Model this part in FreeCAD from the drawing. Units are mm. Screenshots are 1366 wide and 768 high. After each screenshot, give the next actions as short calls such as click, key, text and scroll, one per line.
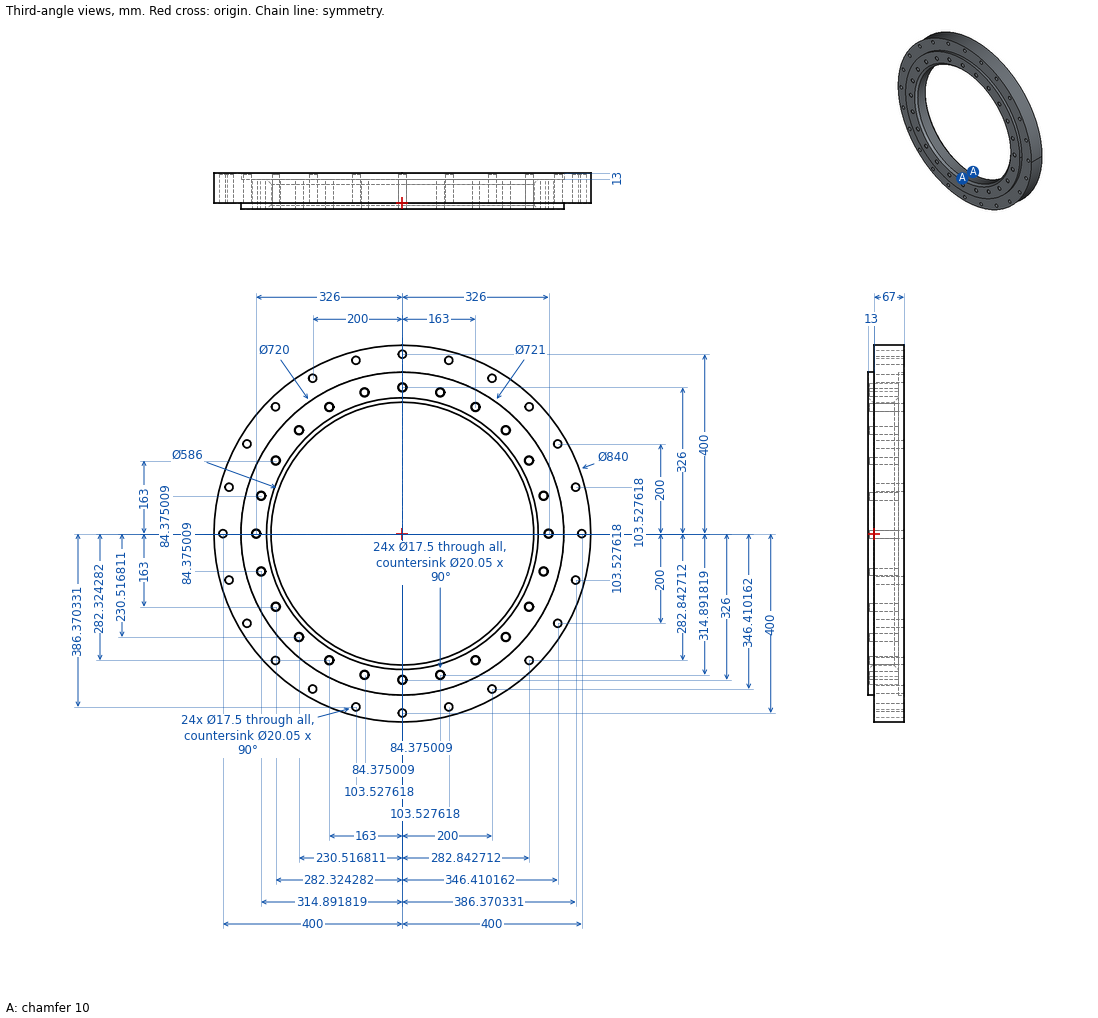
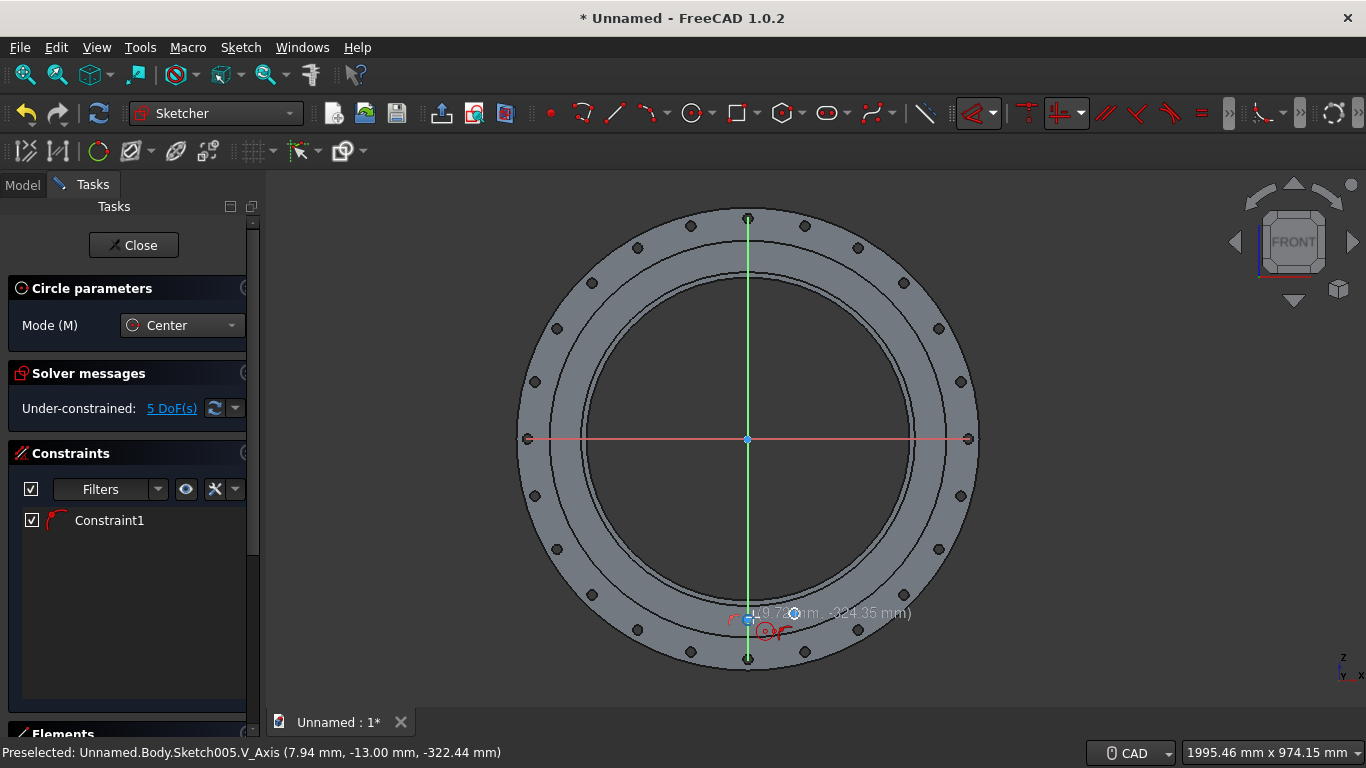
click(701, 613)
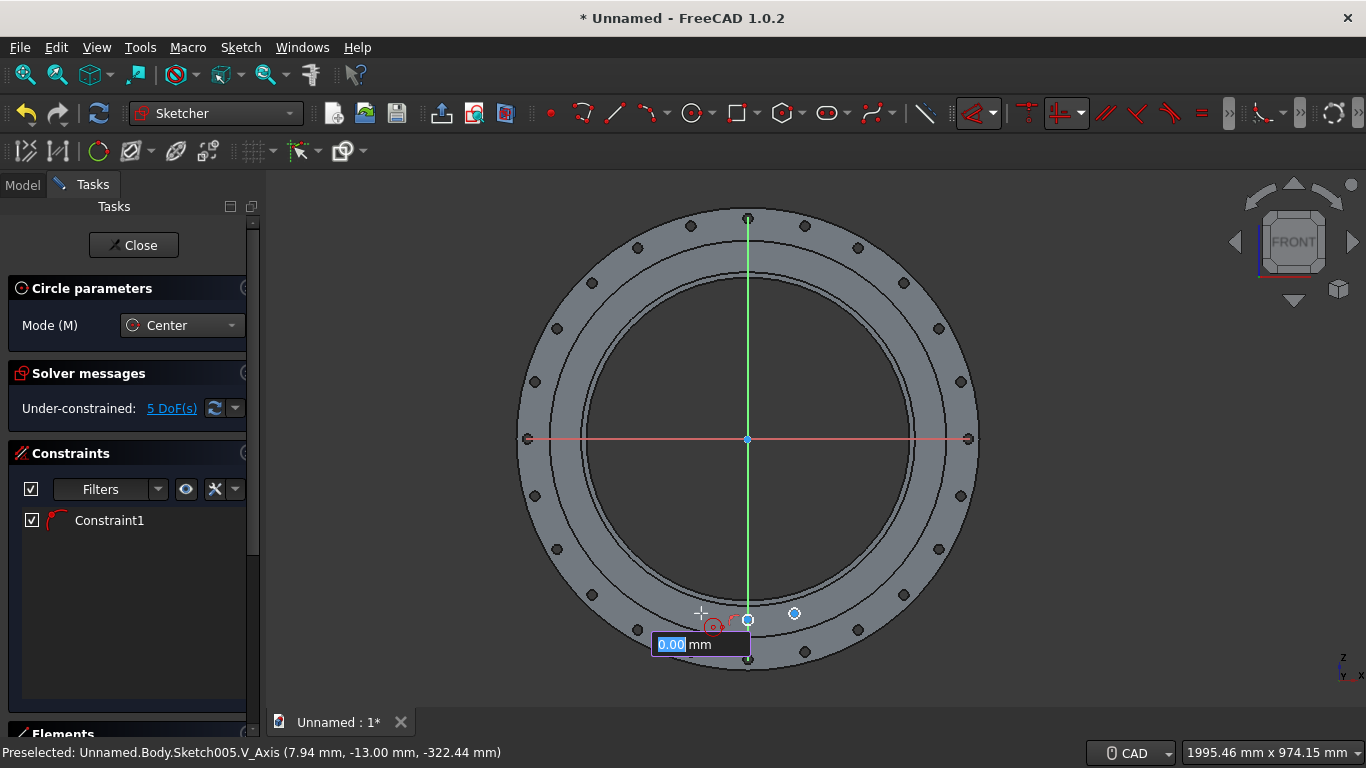
scroll(705, 609, up, 6)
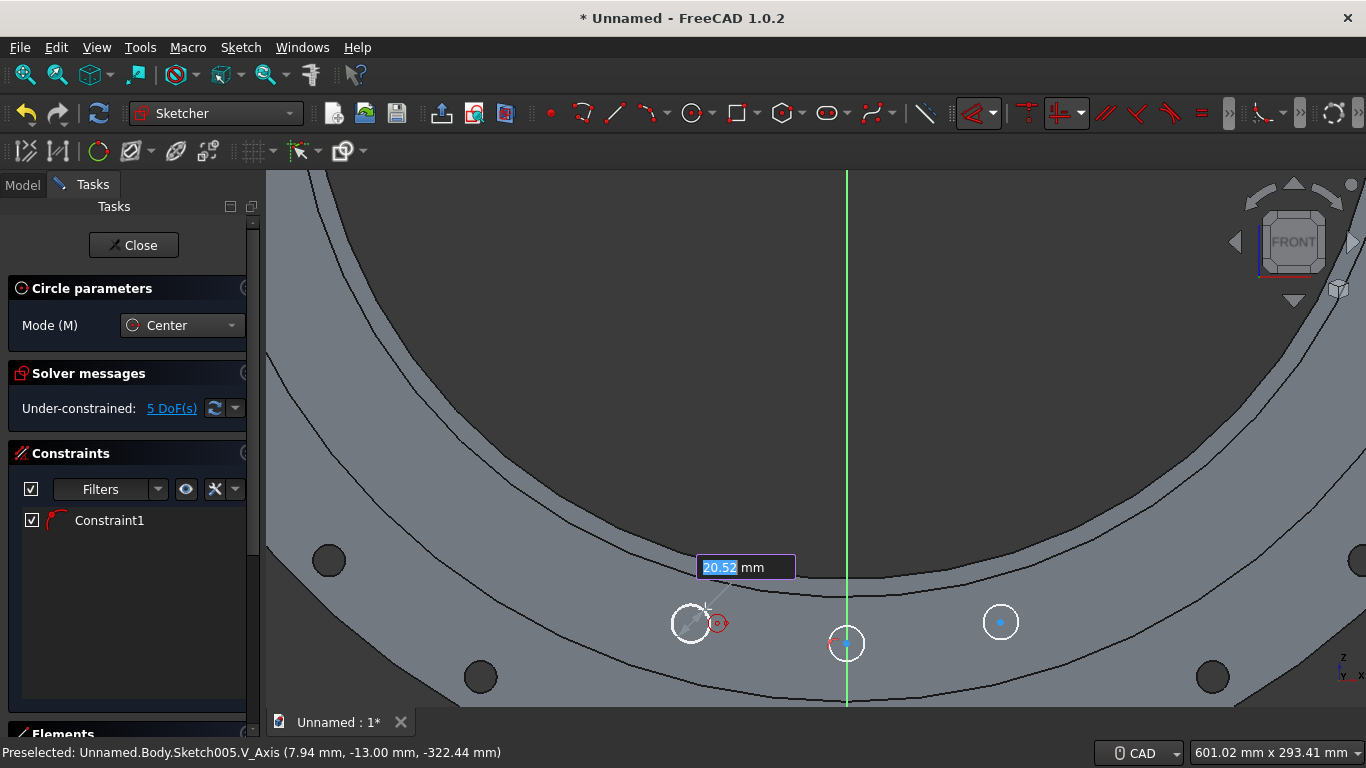
click(704, 608)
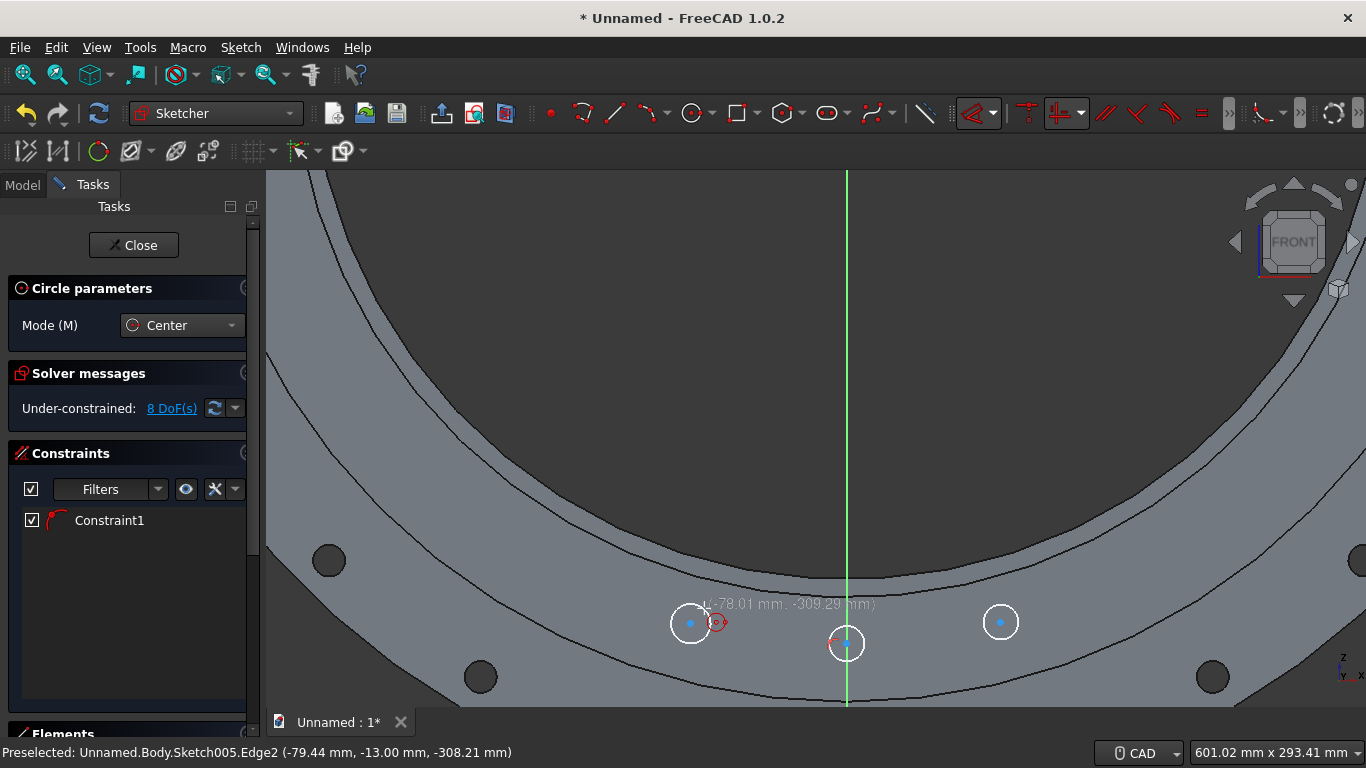
scroll(548, 560, up, 2)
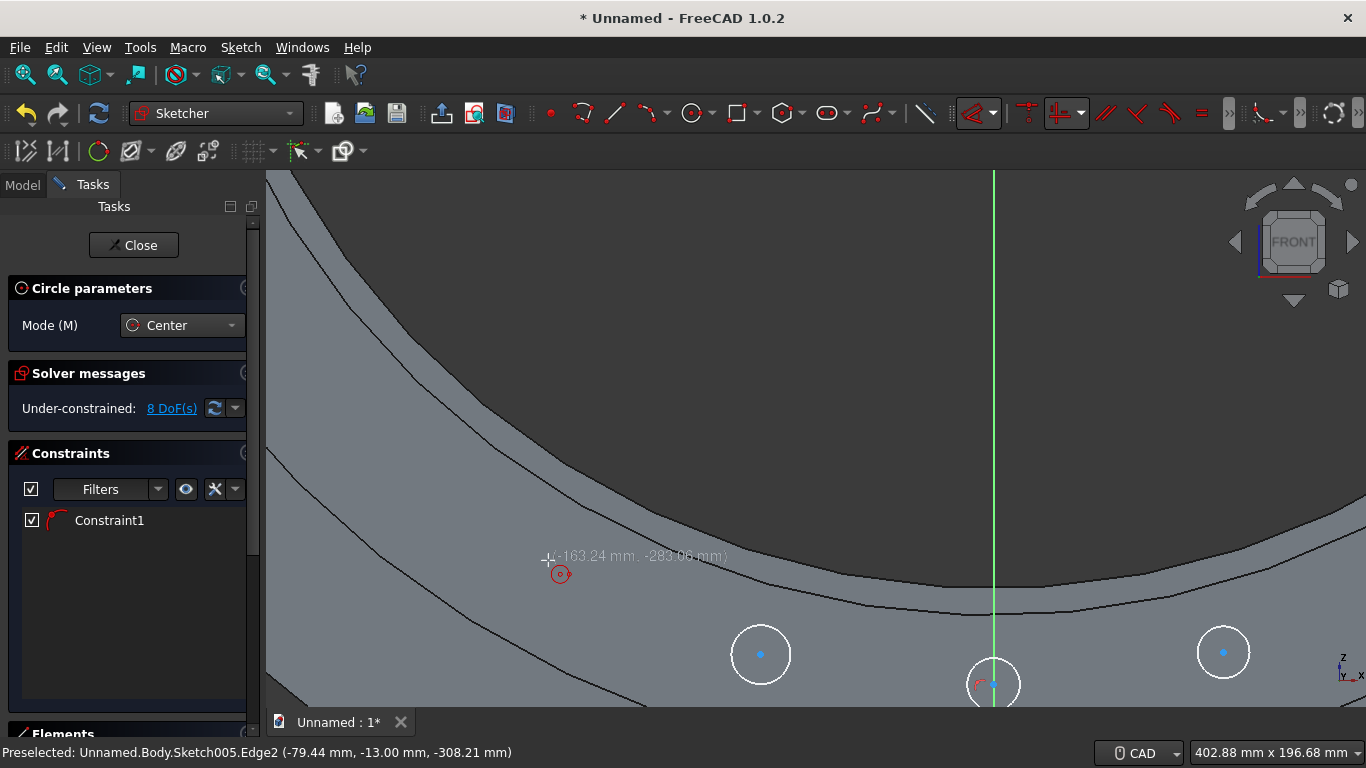
scroll(685, 603, down, 8)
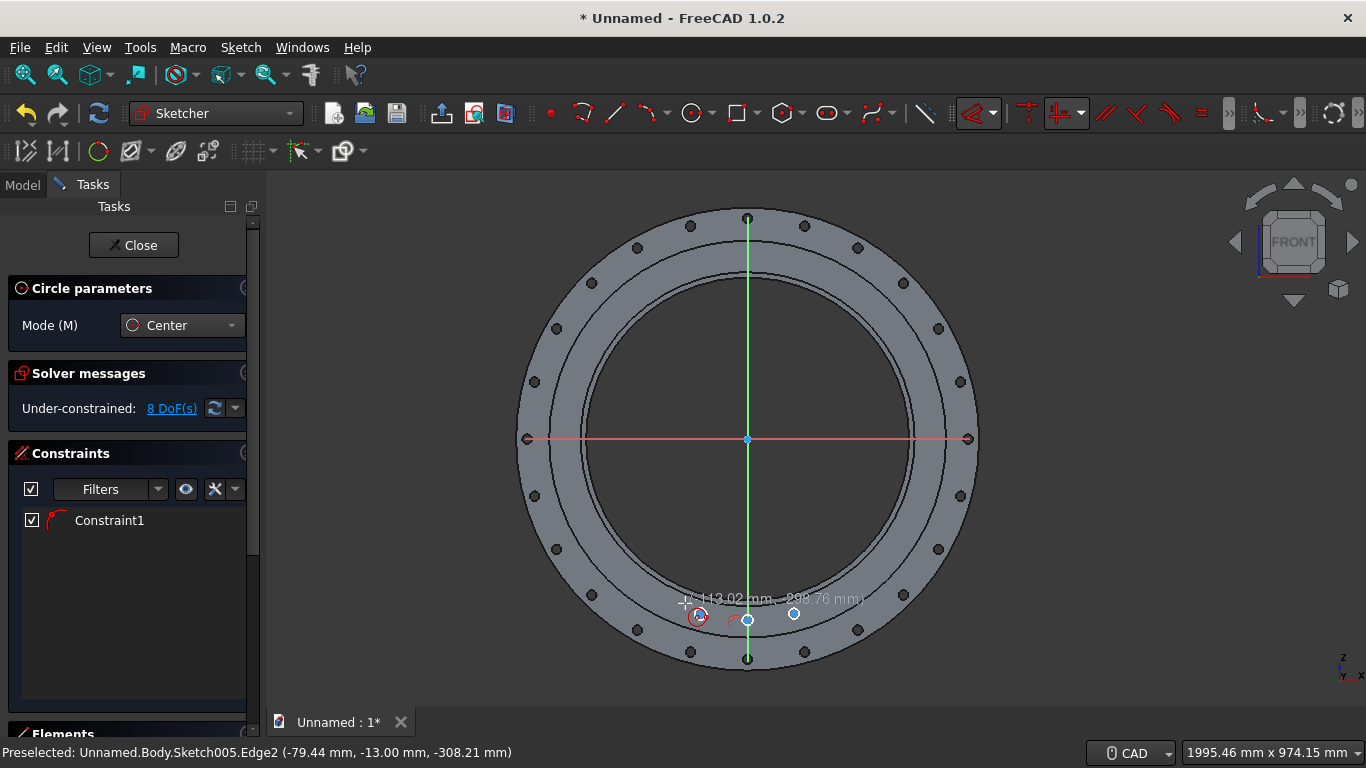
click(658, 595)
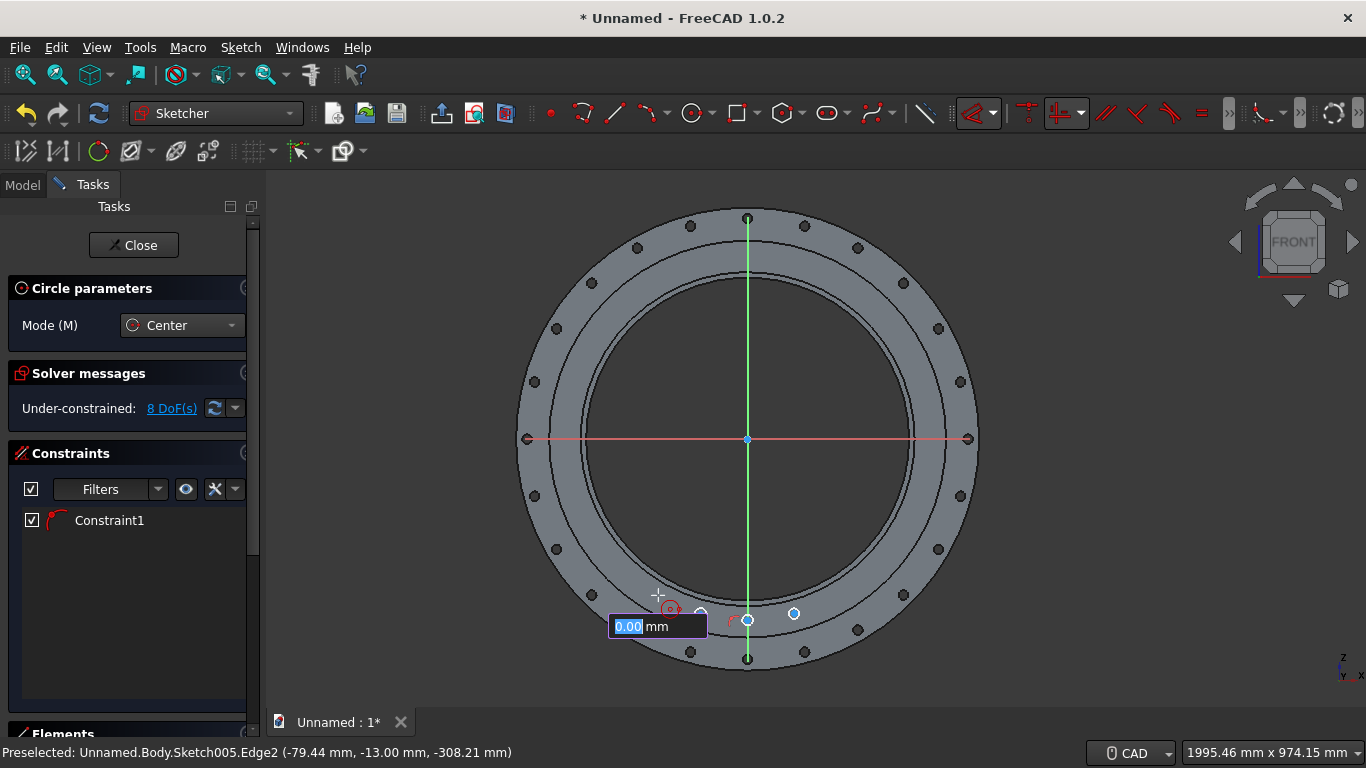
scroll(661, 591, up, 6)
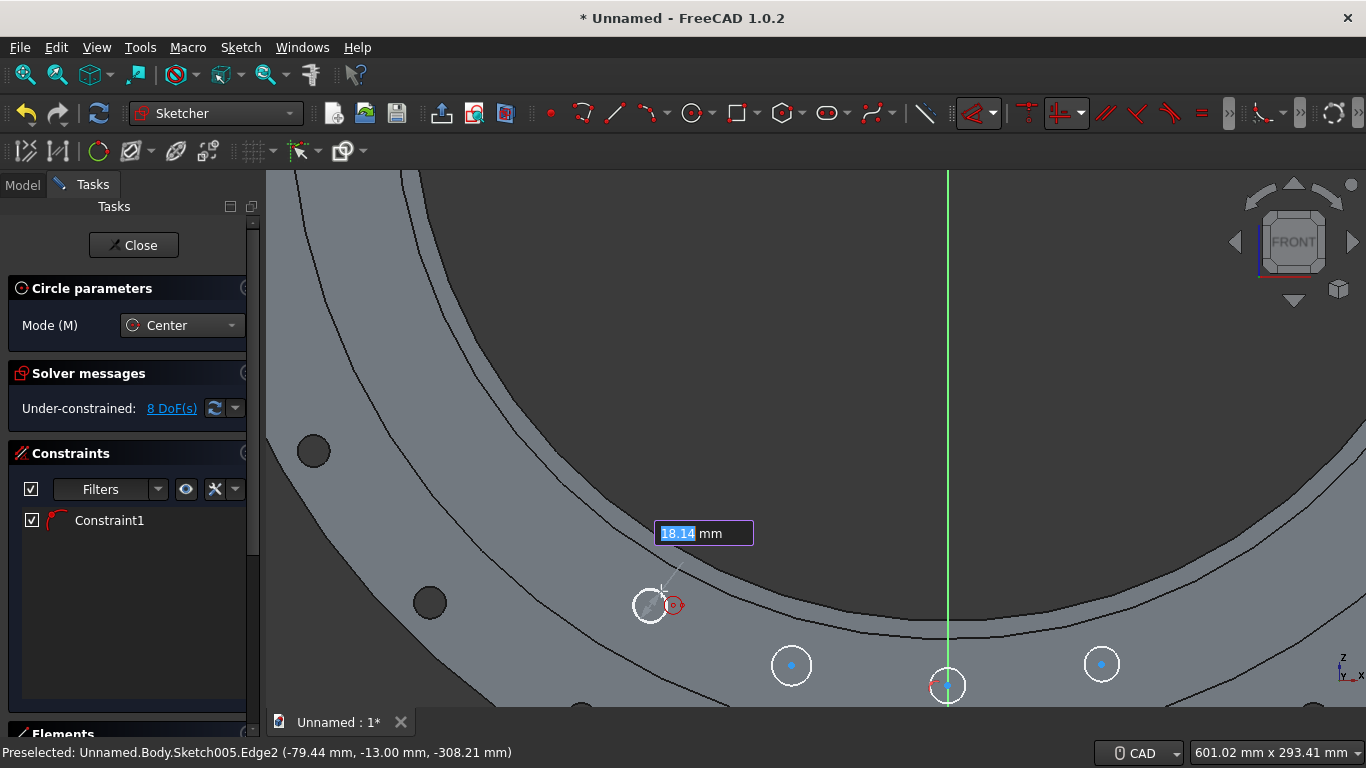
click(661, 590)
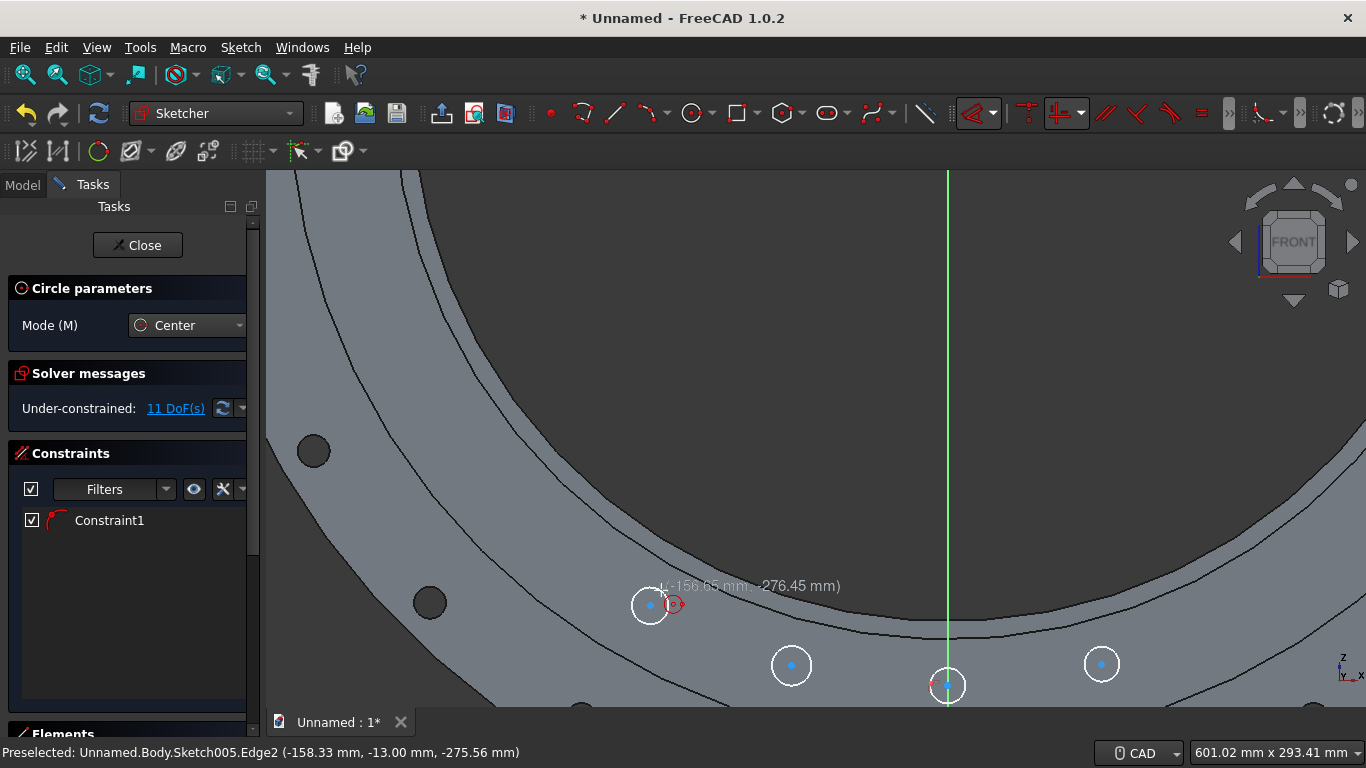
scroll(526, 507, up, 2)